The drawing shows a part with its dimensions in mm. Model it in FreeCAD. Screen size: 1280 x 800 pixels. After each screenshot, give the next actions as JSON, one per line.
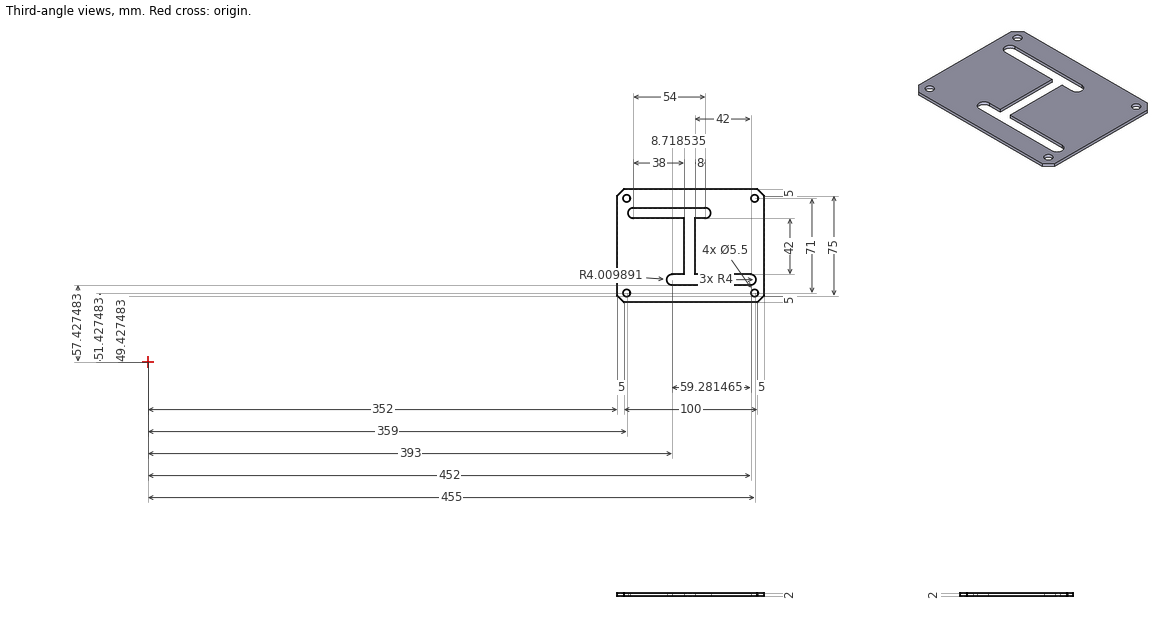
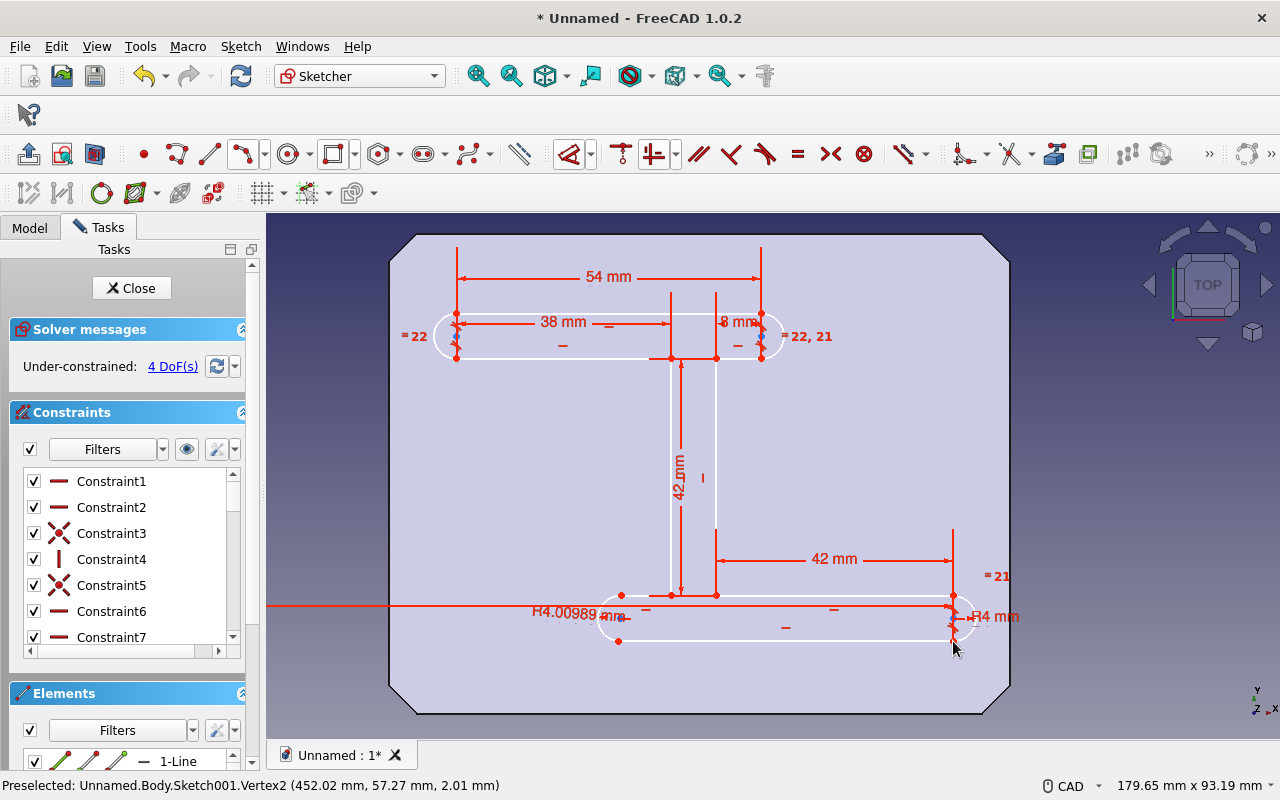
{"action": "left_click", "coordinate": [620, 619]}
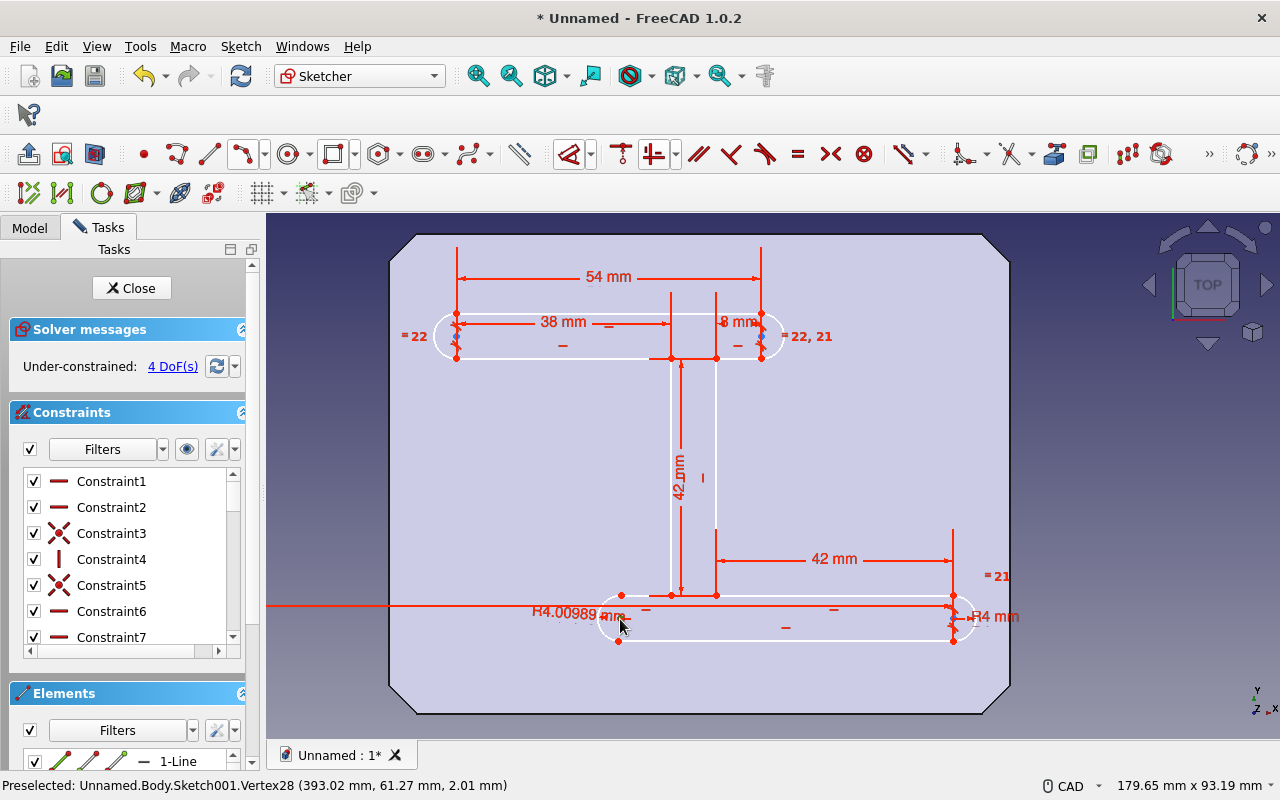
{"action": "left_click", "coordinate": [590, 154]}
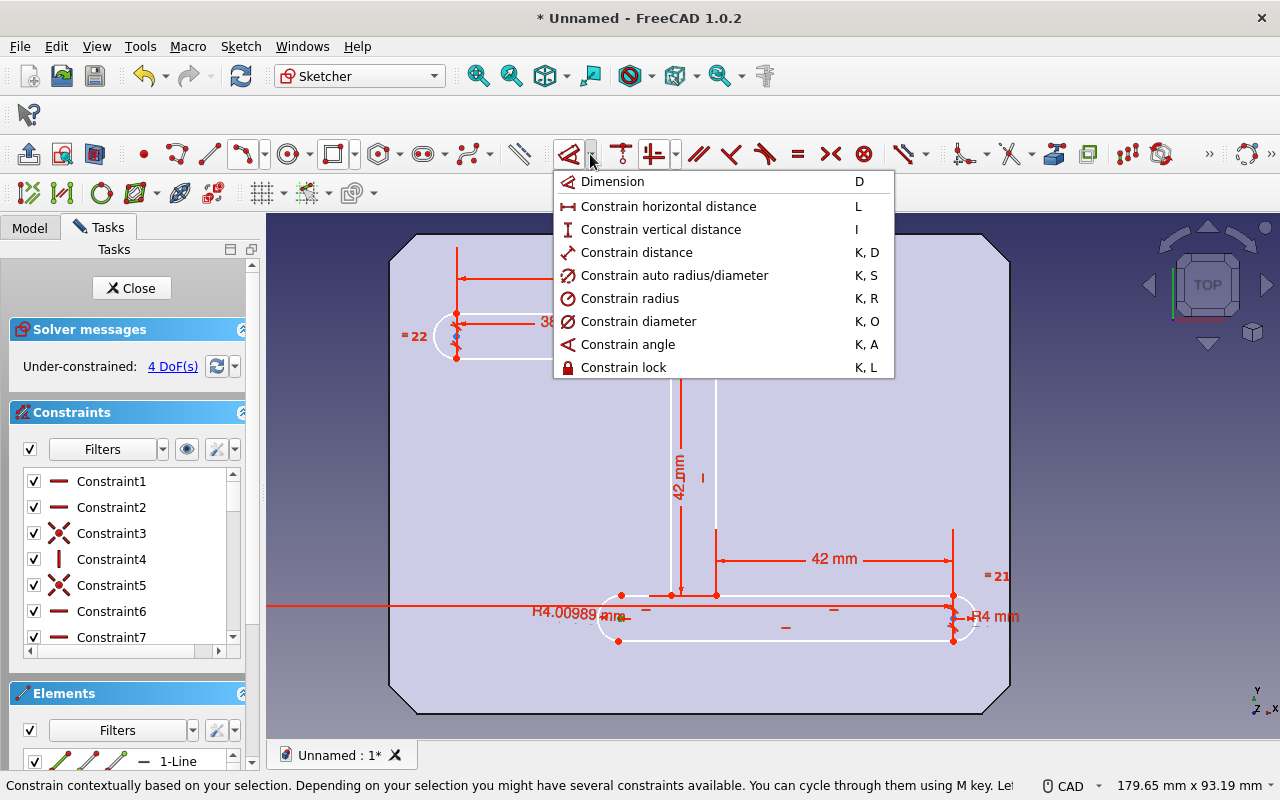
{"action": "left_click", "coordinate": [724, 206]}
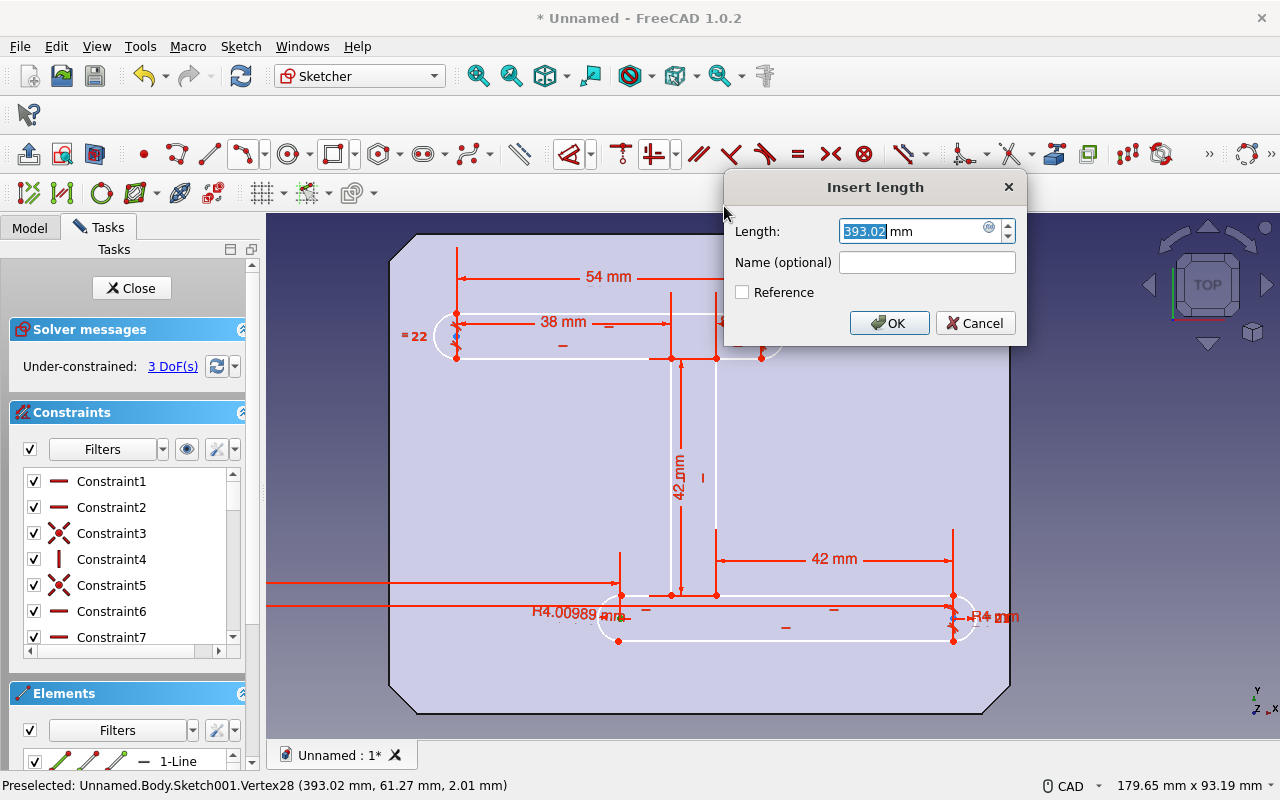
{"action": "type", "text": "393"}
{"action": "key", "text": "Return"}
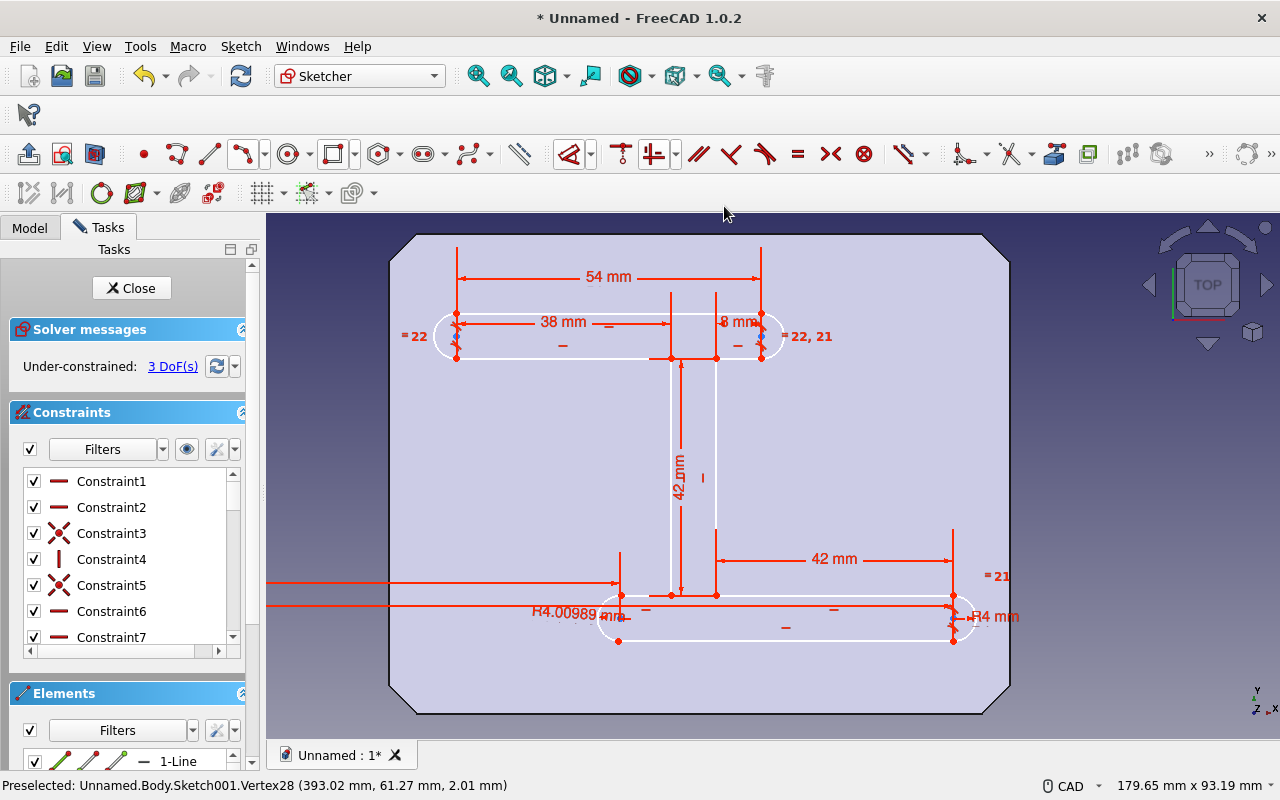
{"action": "left_click", "coordinate": [656, 596]}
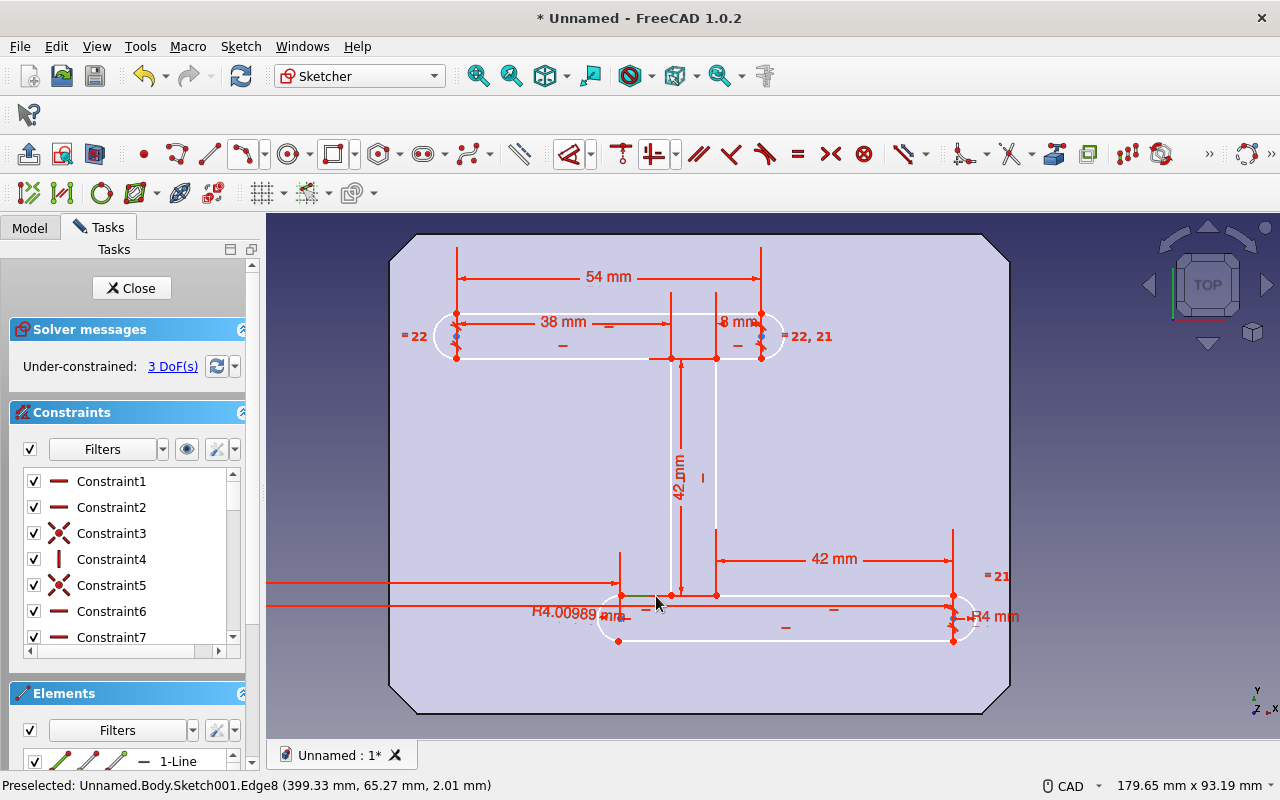
{"action": "key", "text": "l"}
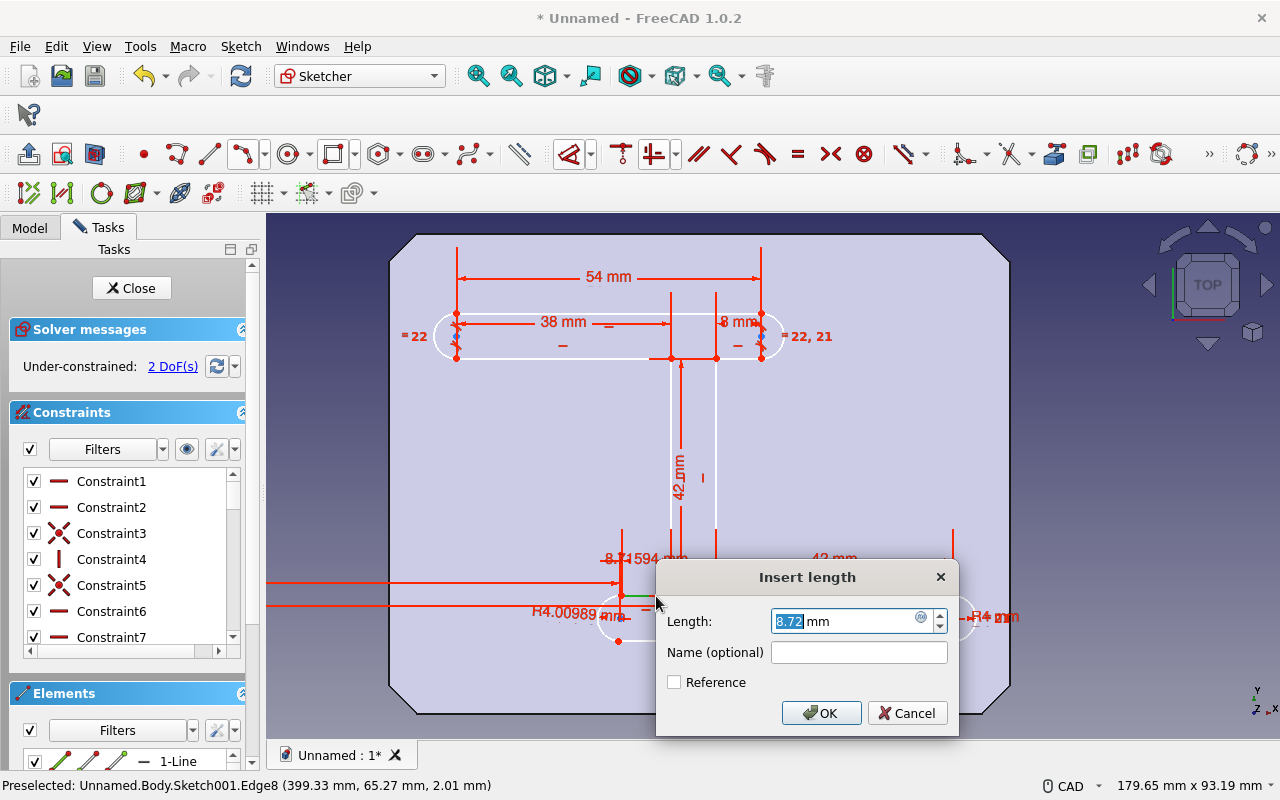
{"action": "type", "text": "8.718535"}
{"action": "key", "text": "Return"}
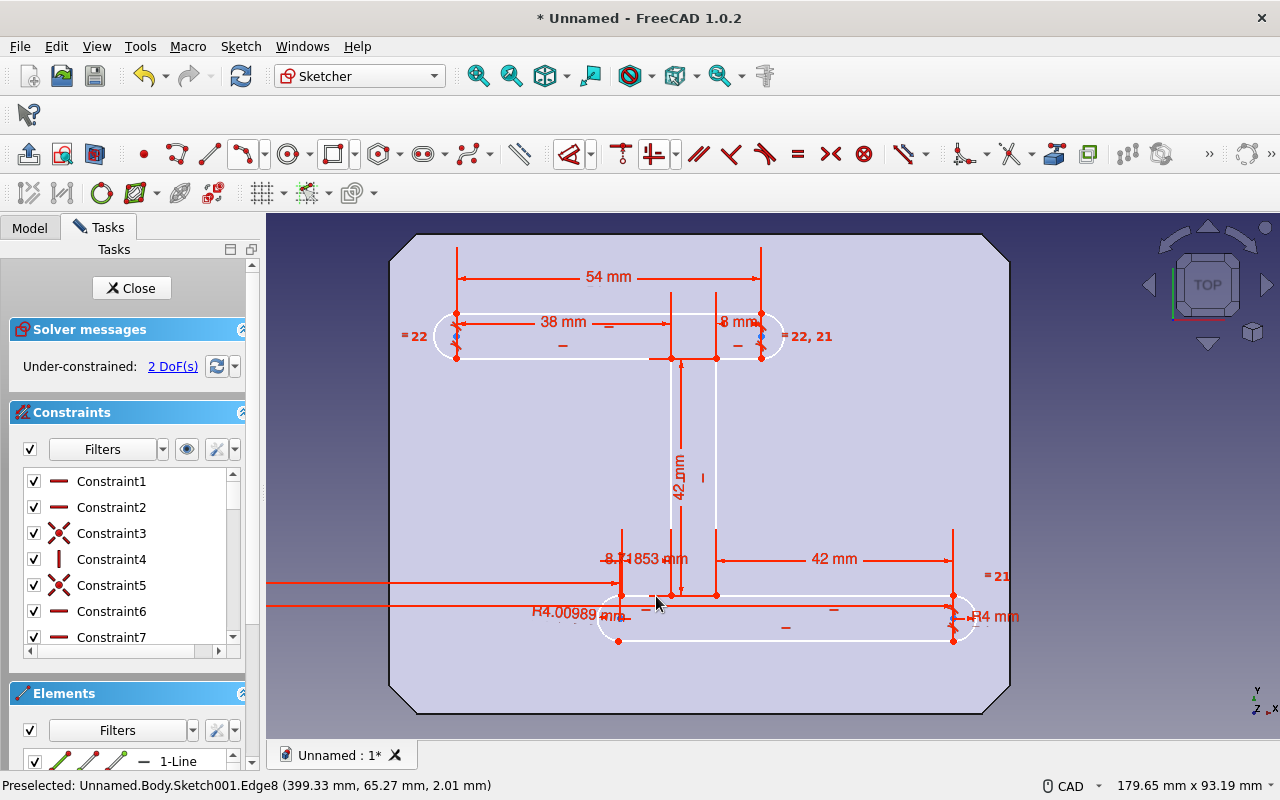
{"action": "left_click", "coordinate": [719, 641]}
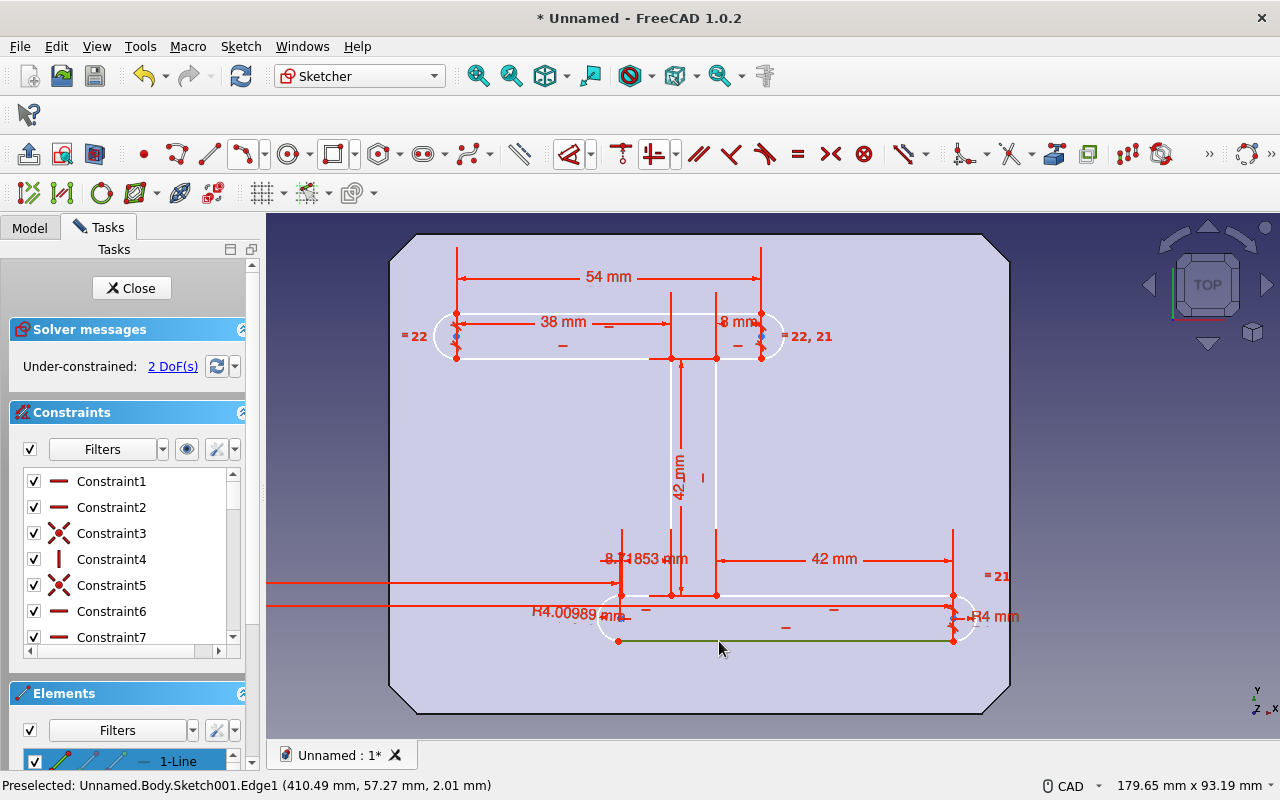
{"action": "key", "text": "l"}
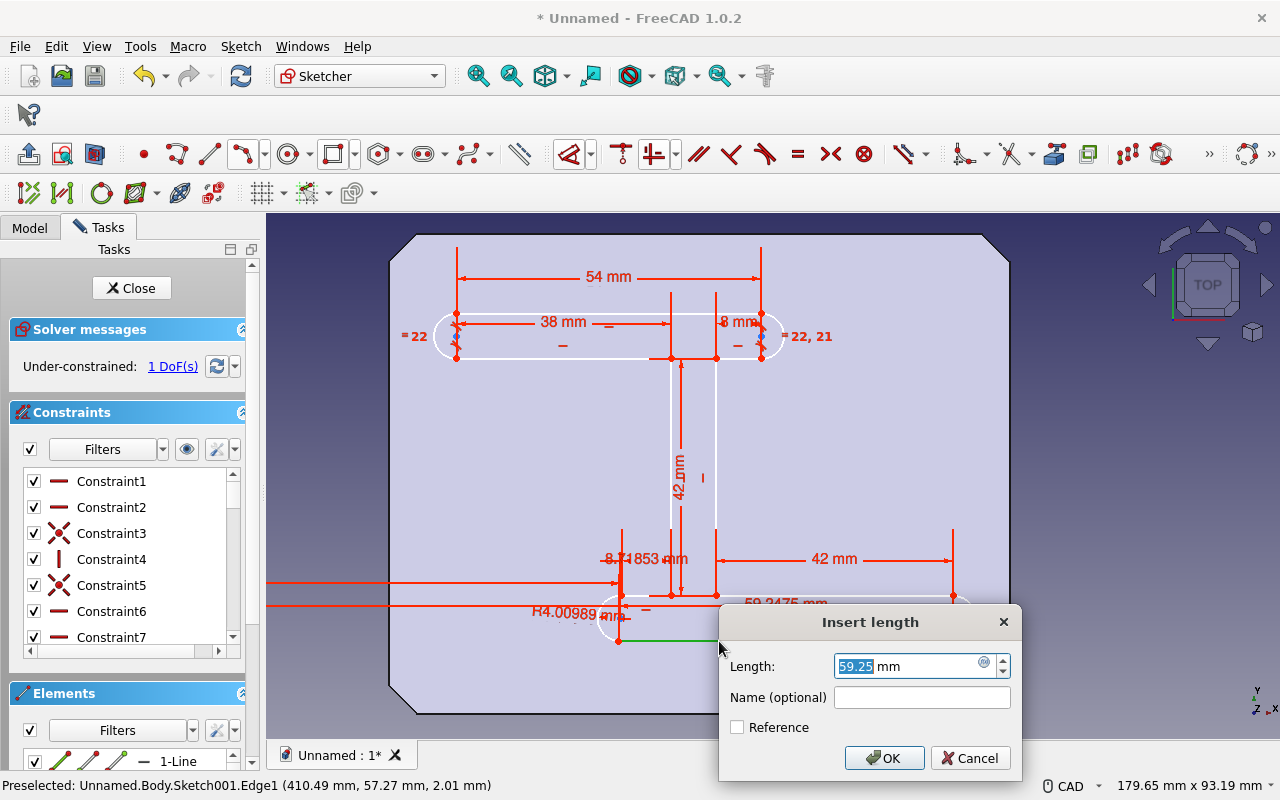
{"action": "type", "text": "59.281465"}
{"action": "key", "text": "Return"}